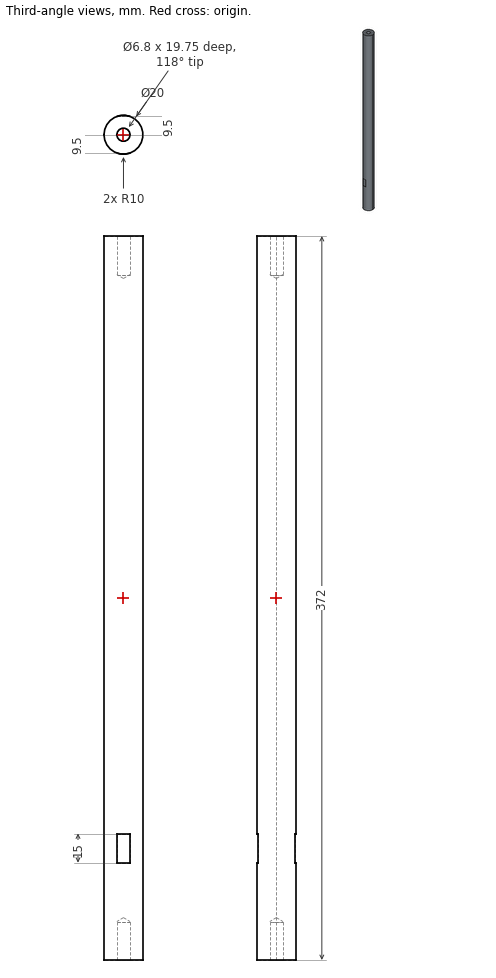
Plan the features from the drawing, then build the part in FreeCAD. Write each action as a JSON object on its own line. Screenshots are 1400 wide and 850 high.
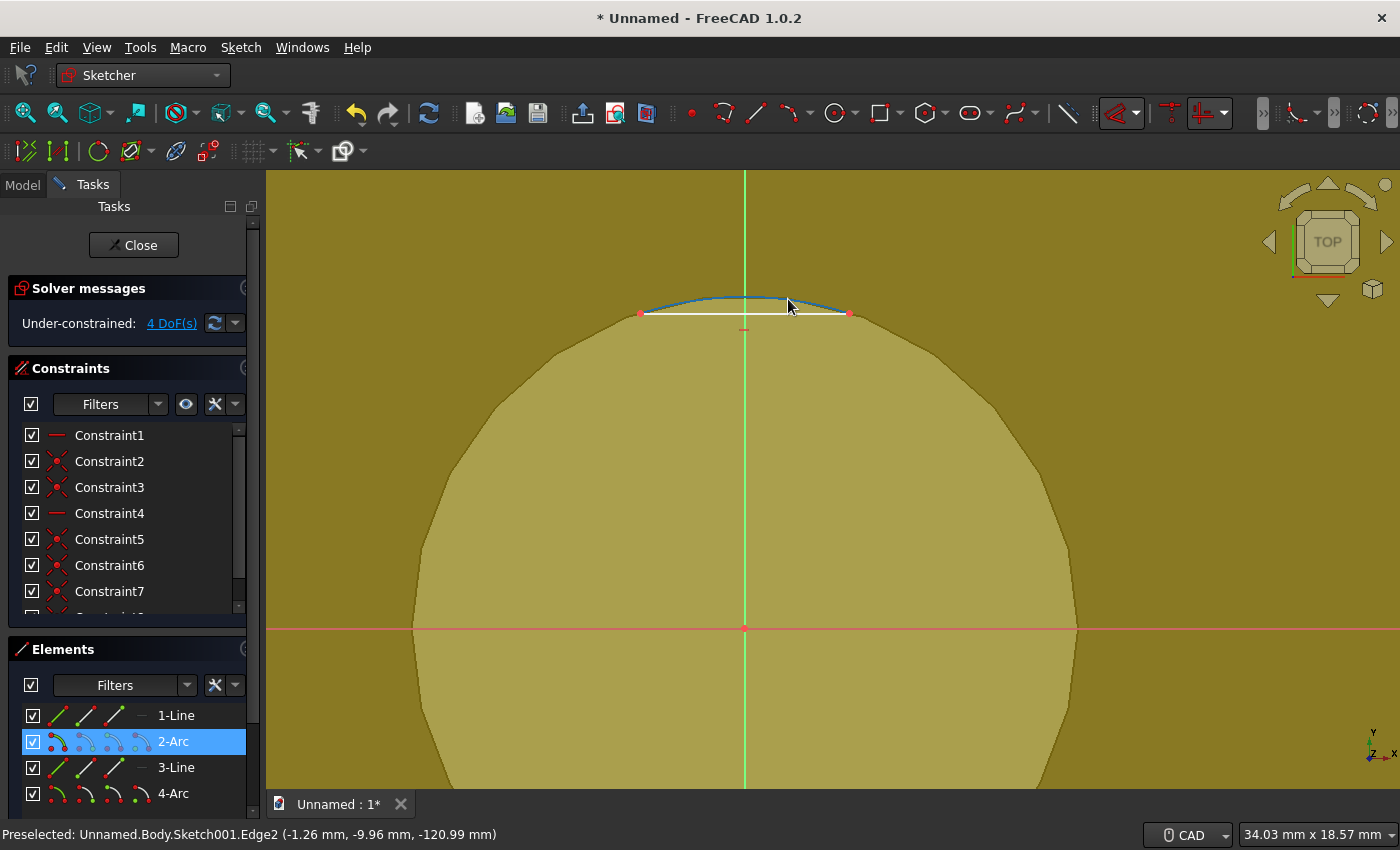
{"action": "left_click", "coordinate": [787, 300]}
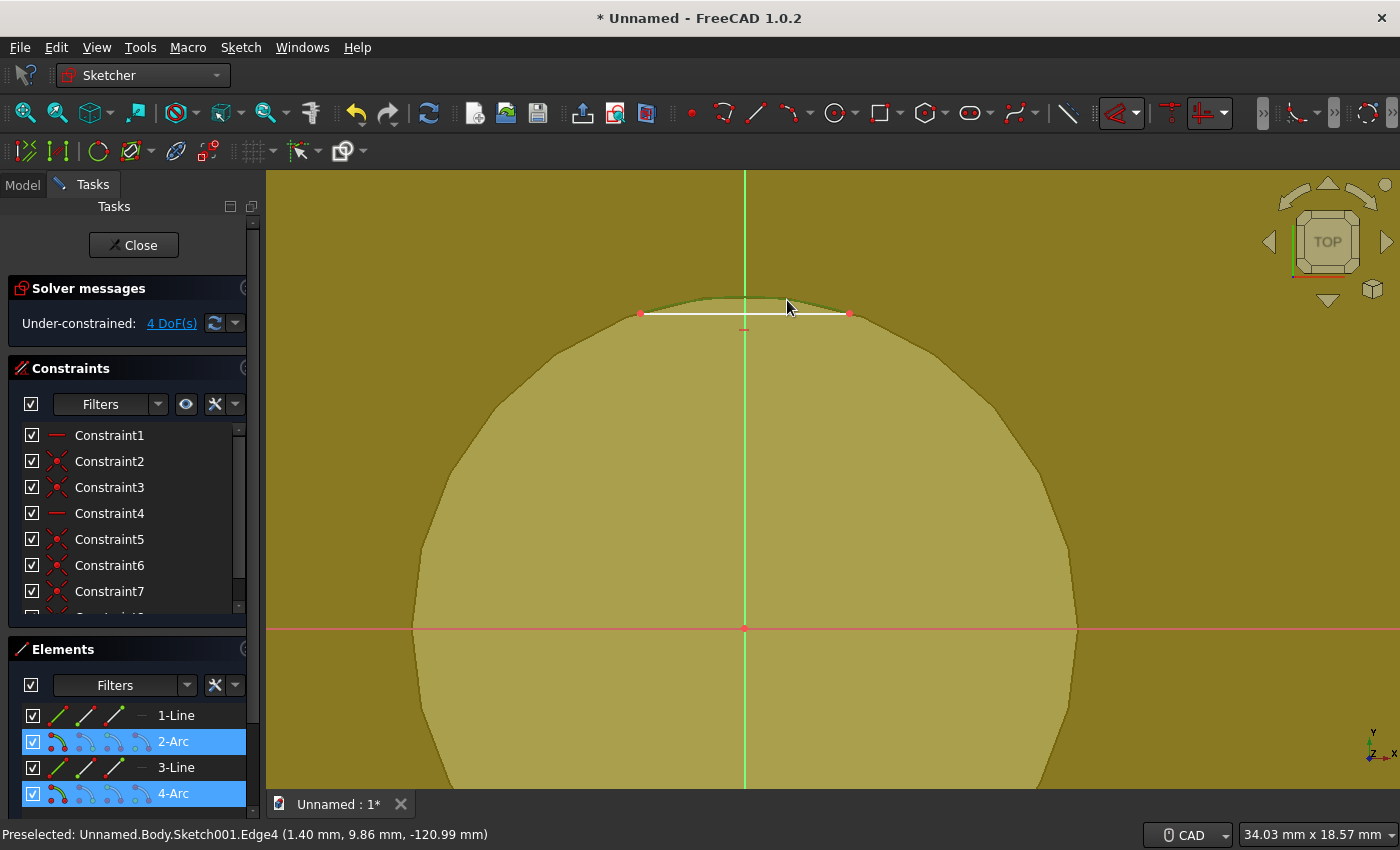
{"action": "key", "text": "e"}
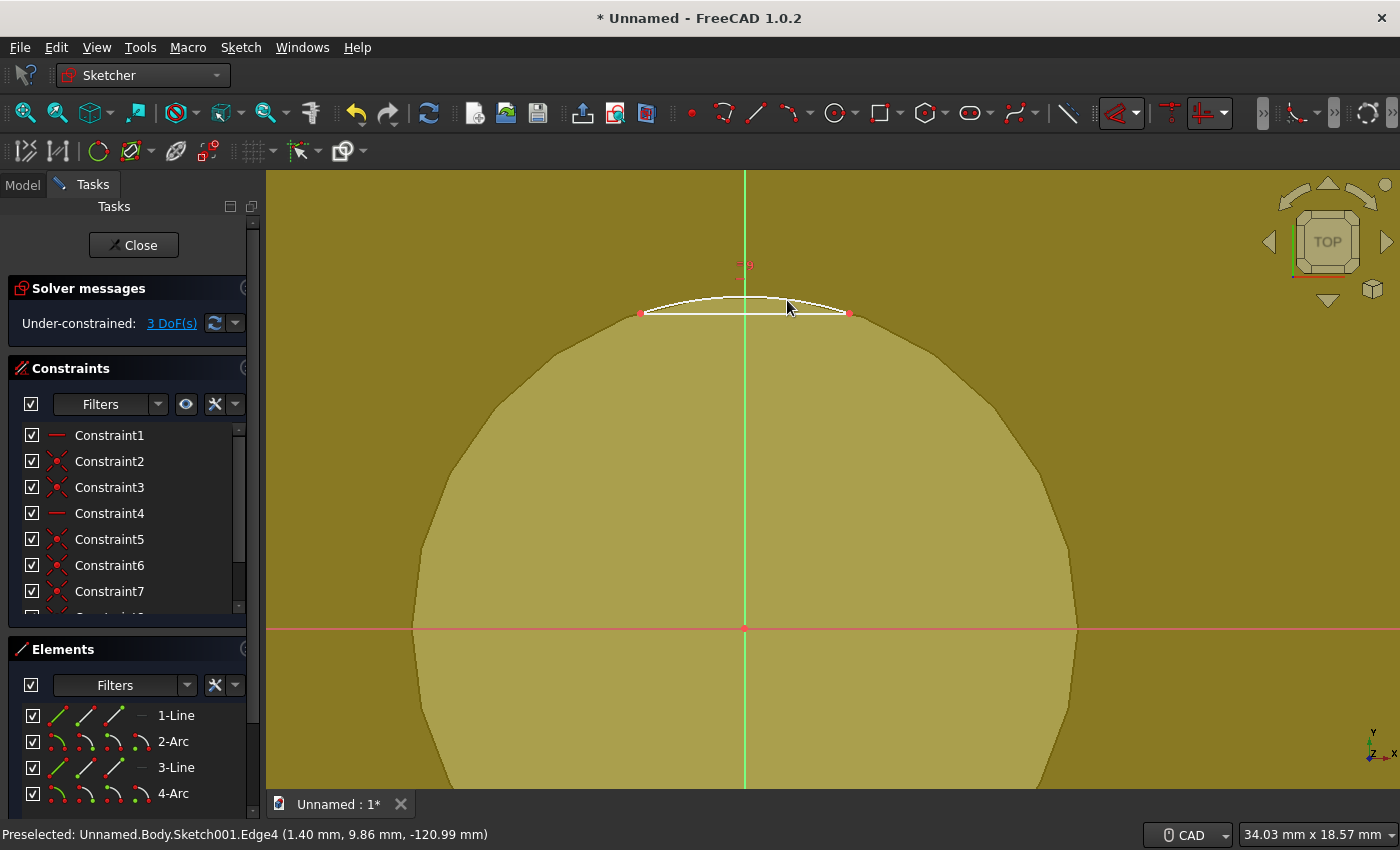
{"action": "scroll", "coordinate": [788, 298], "scroll_direction": "down", "scroll_amount": 3}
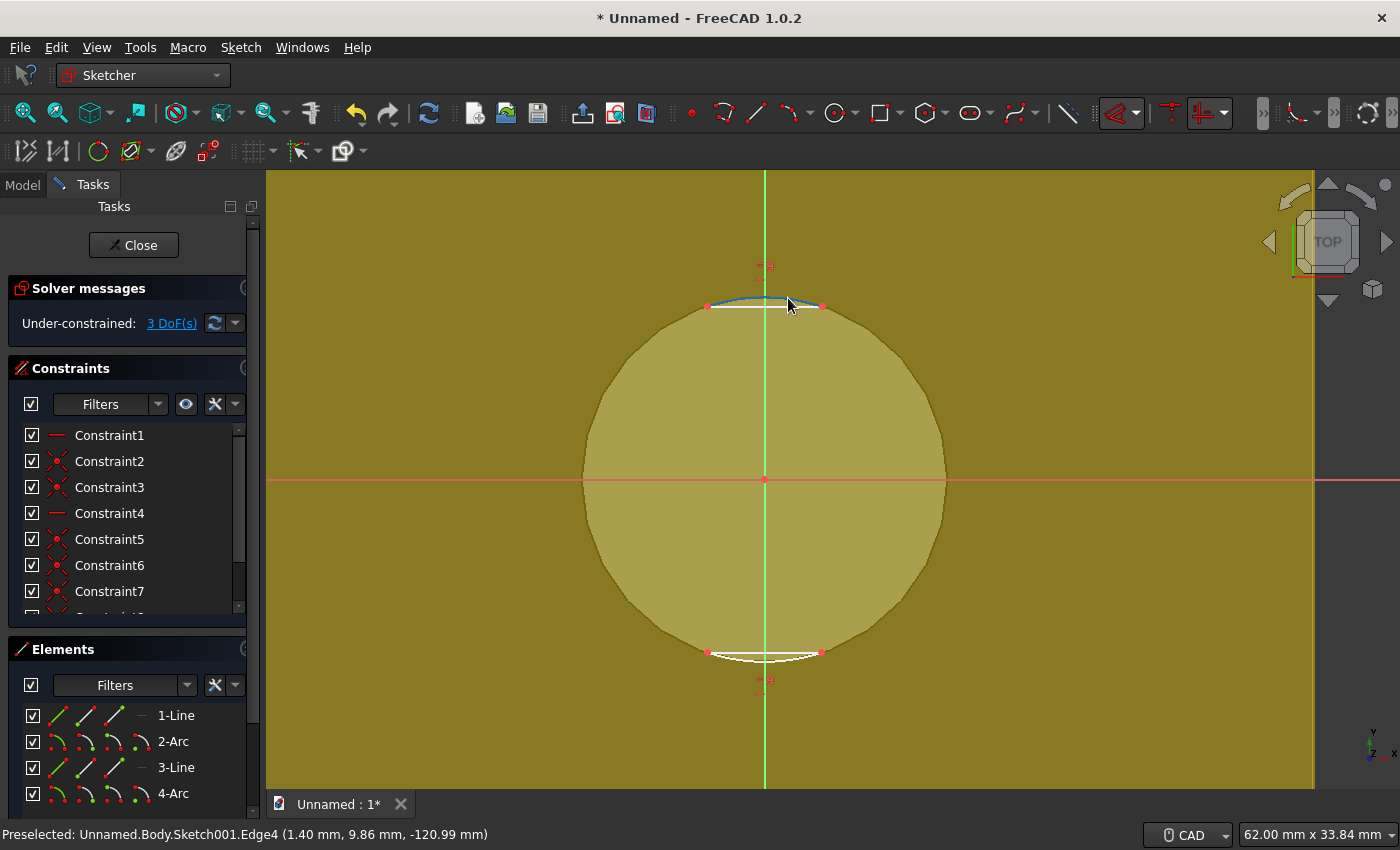
{"action": "scroll", "coordinate": [742, 660], "scroll_direction": "up", "scroll_amount": 3}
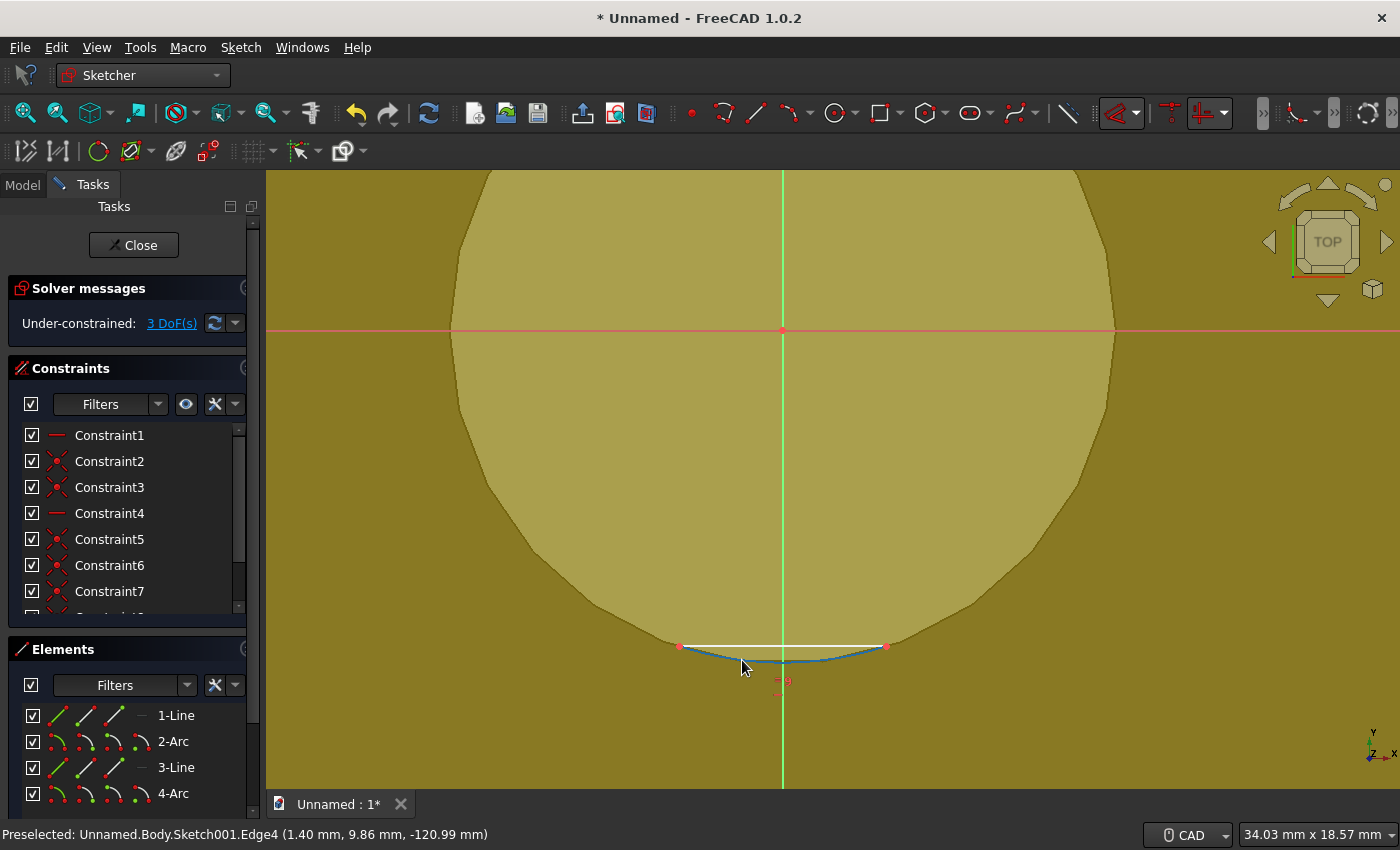
{"action": "left_click", "coordinate": [741, 660]}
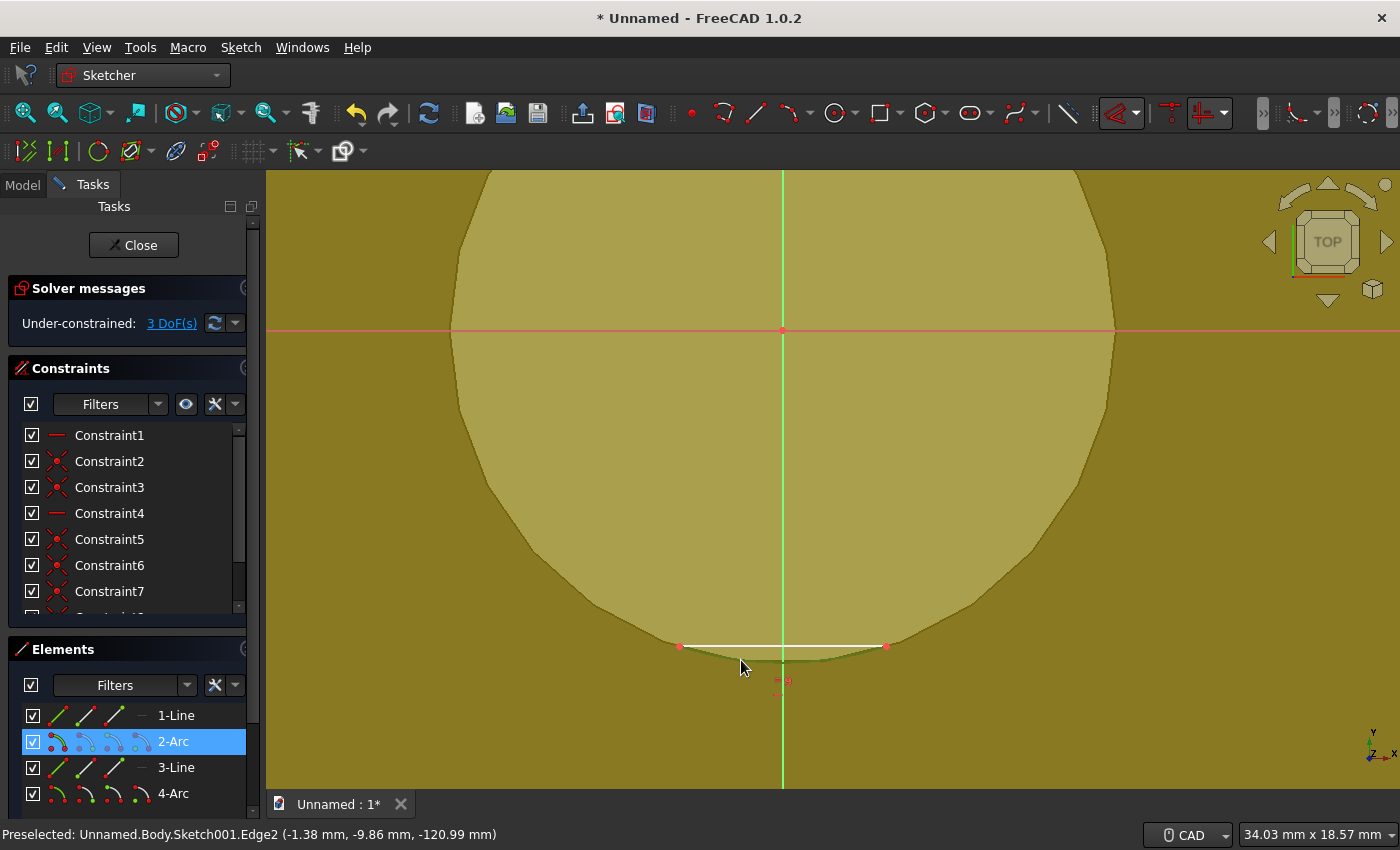
{"action": "left_click", "coordinate": [1138, 114]}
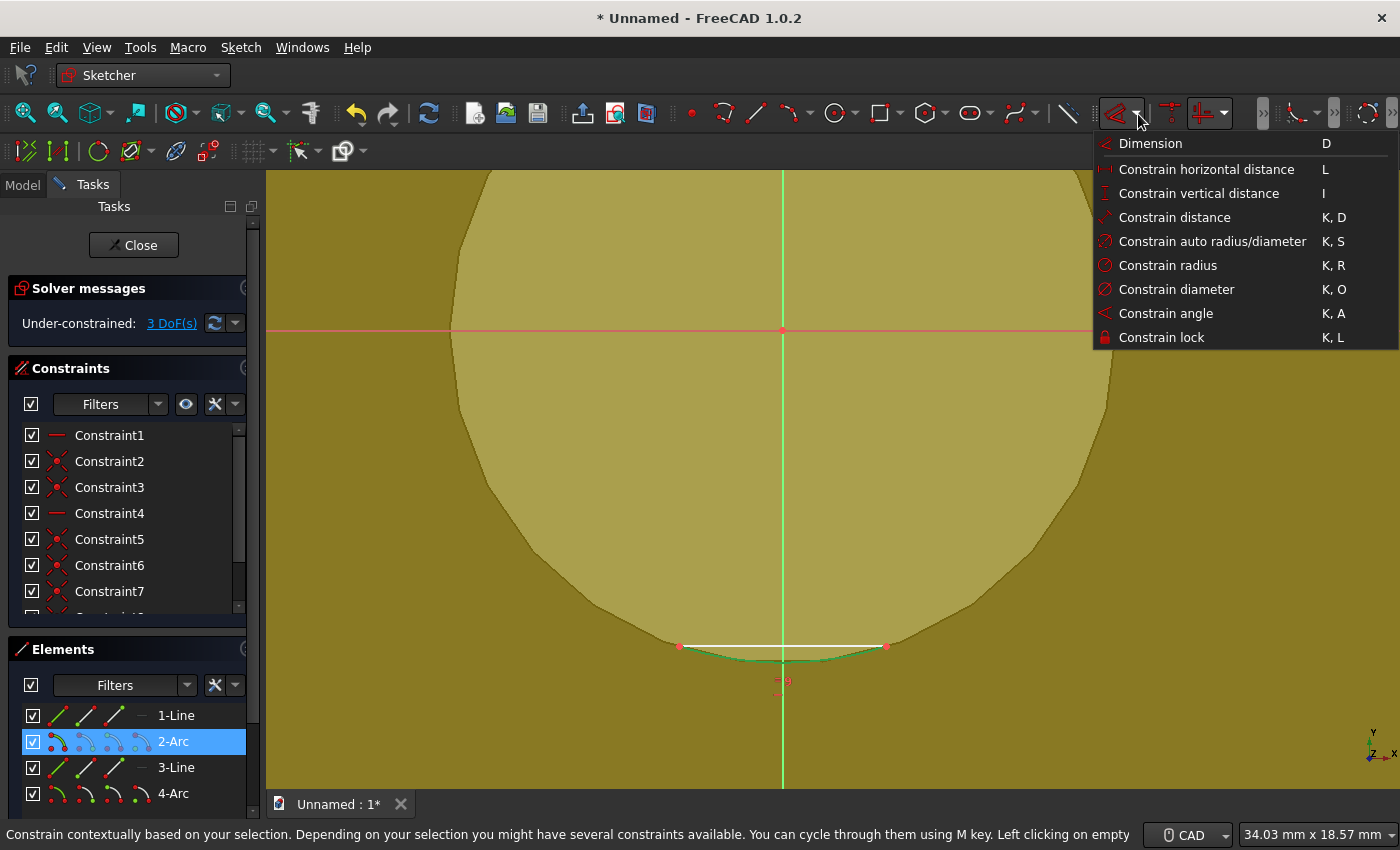
{"action": "left_click", "coordinate": [1246, 265]}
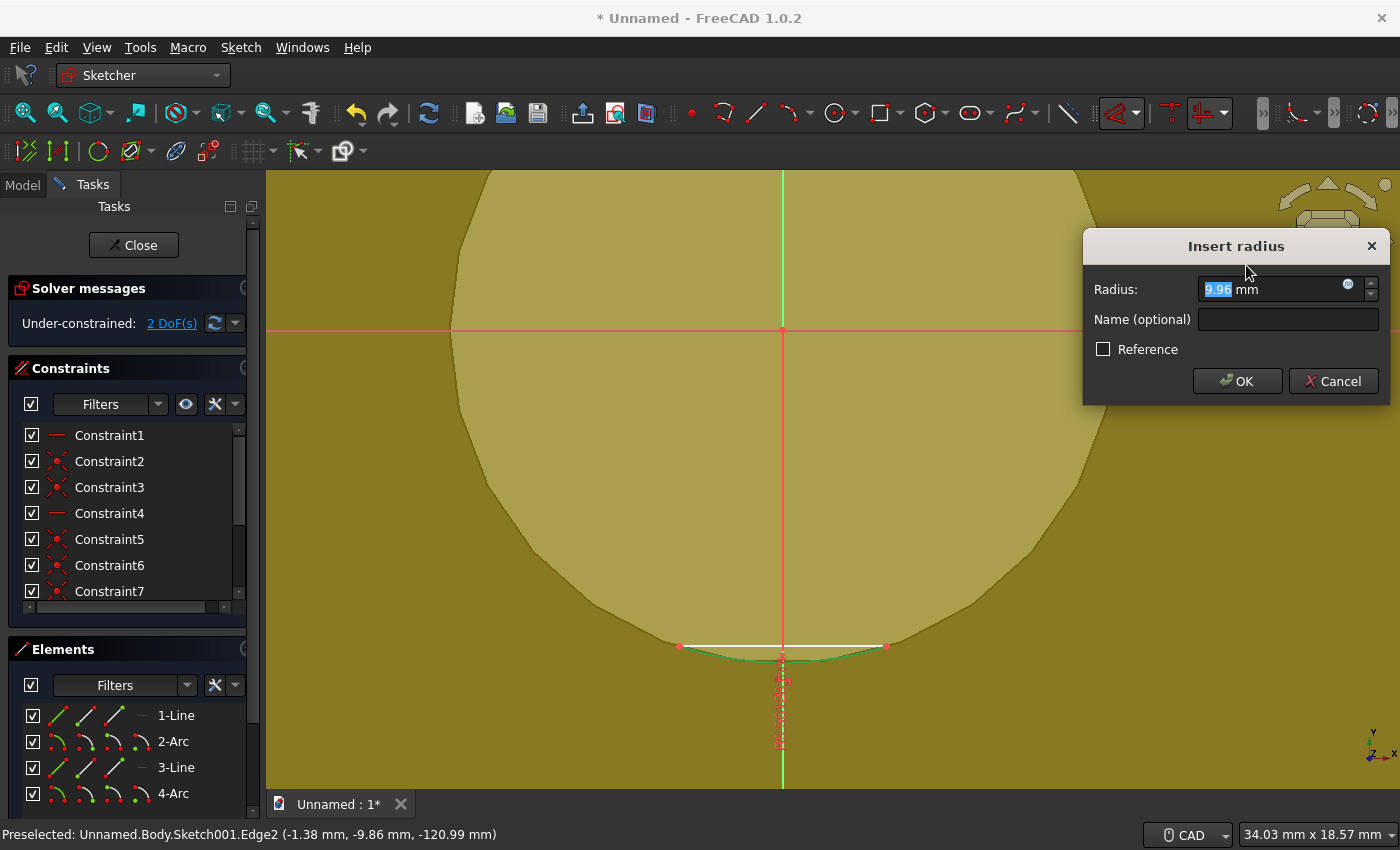
{"action": "type", "text": "10"}
{"action": "key", "text": "Return"}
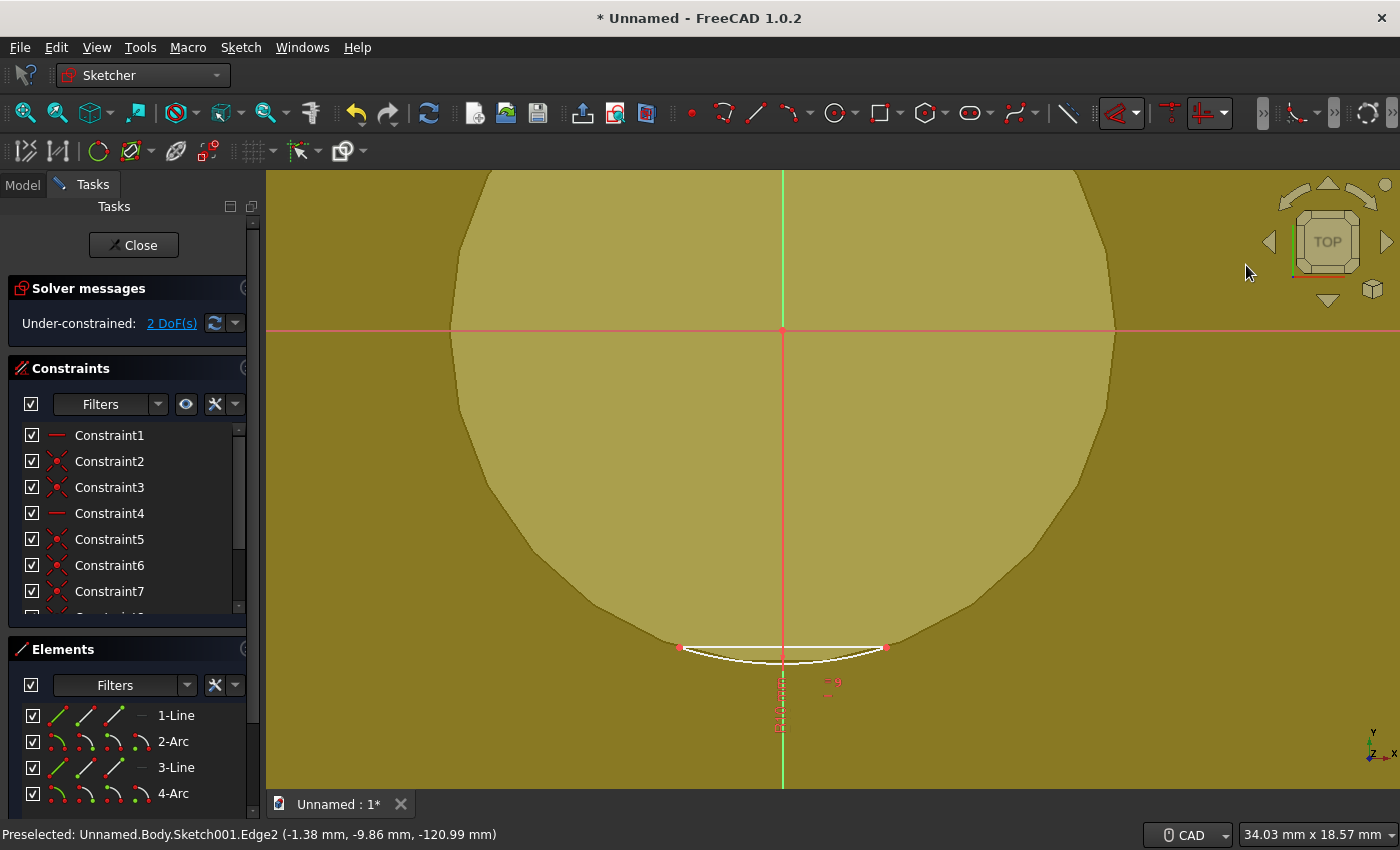
{"action": "left_click", "coordinate": [679, 647]}